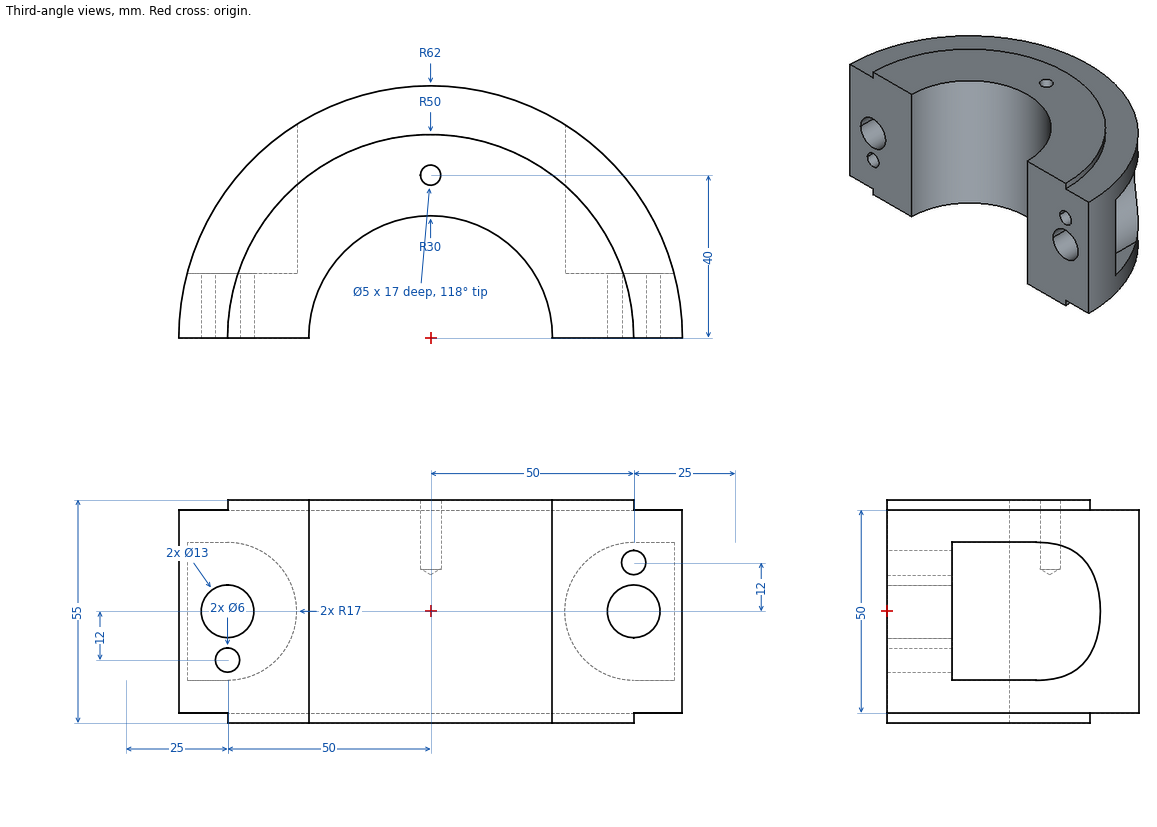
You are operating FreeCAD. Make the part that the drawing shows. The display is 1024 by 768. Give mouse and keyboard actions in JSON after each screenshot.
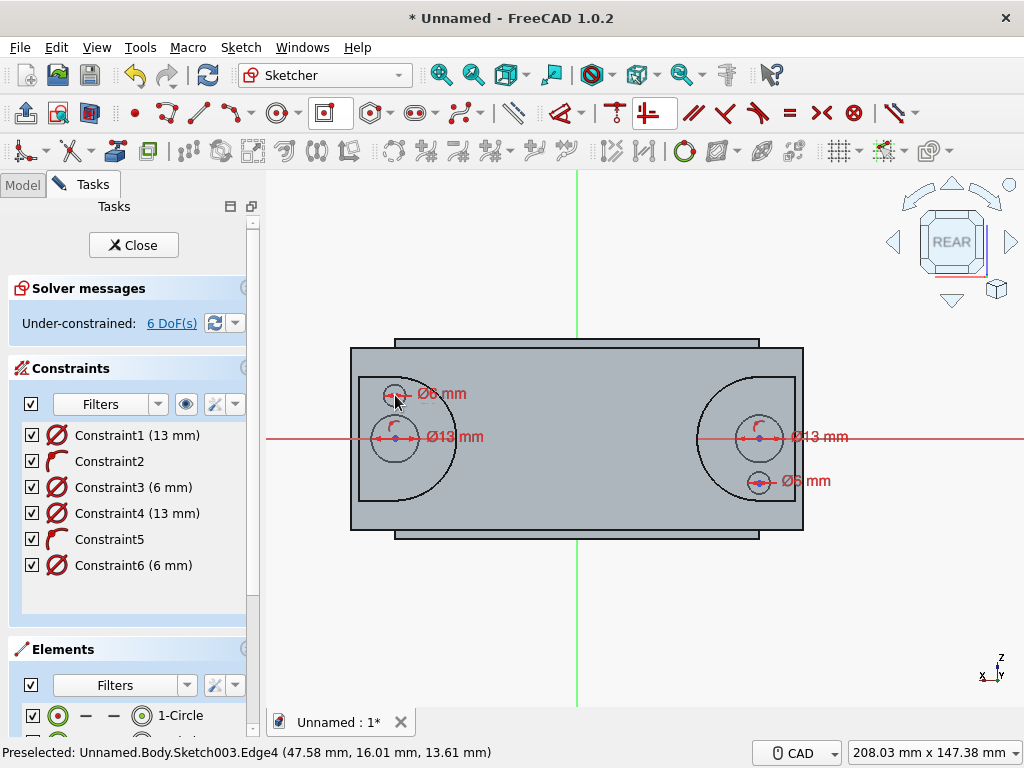
{"action": "left_click", "coordinate": [760, 439]}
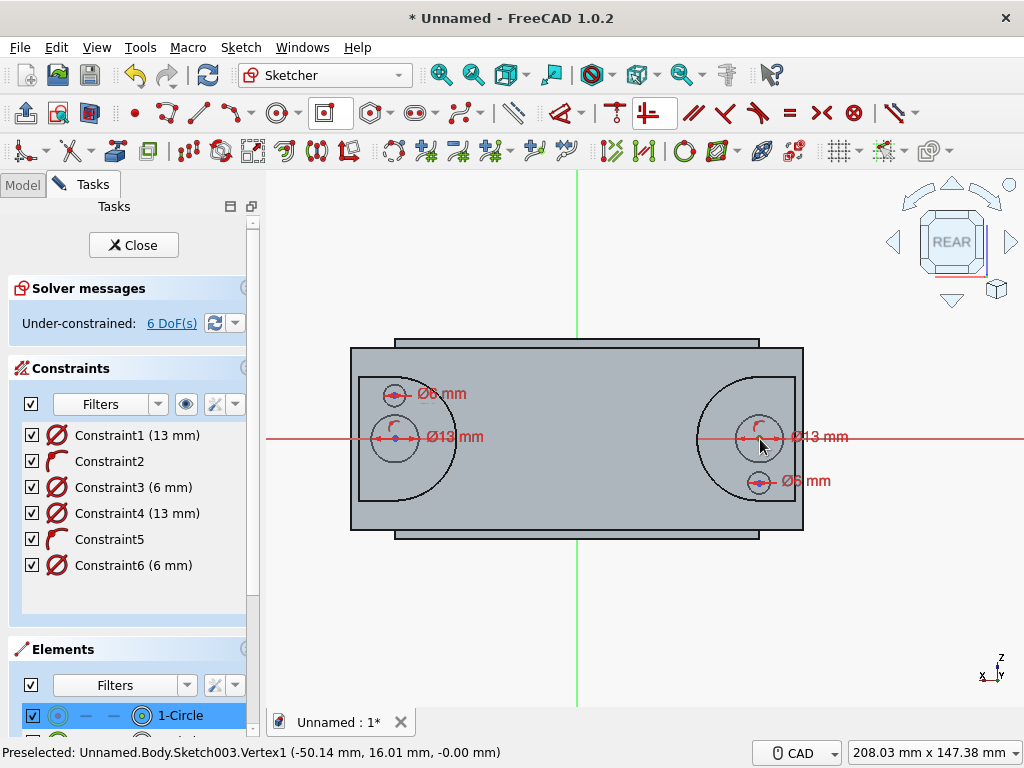
{"action": "left_click", "coordinate": [759, 483]}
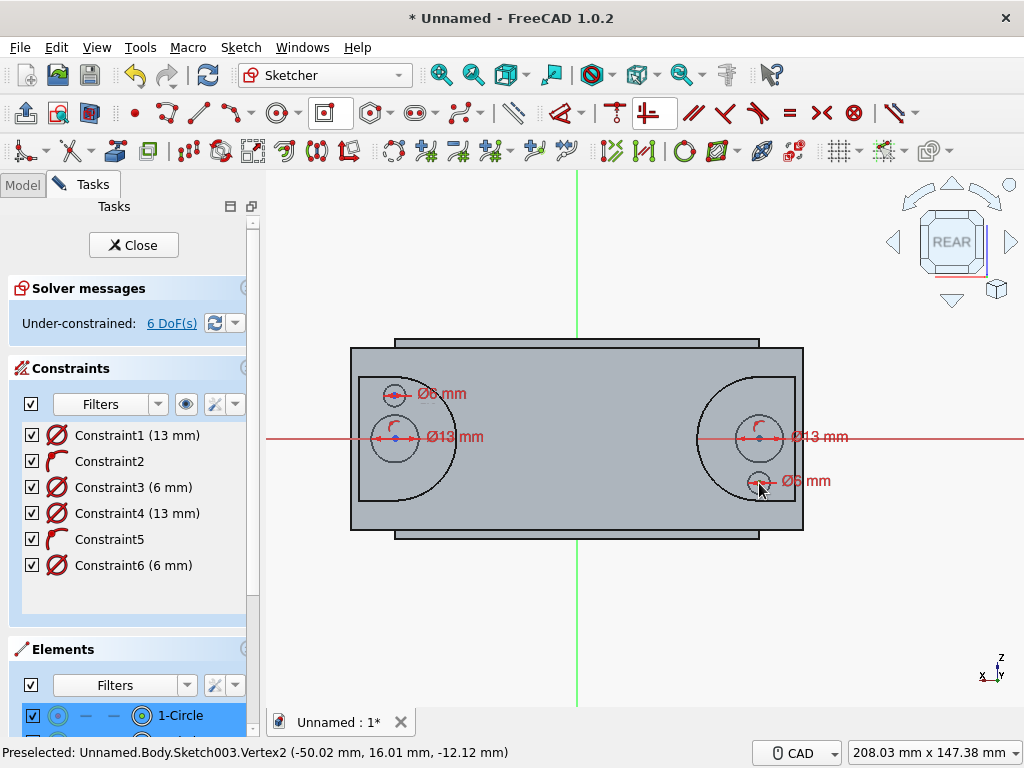
{"action": "key", "text": "v"}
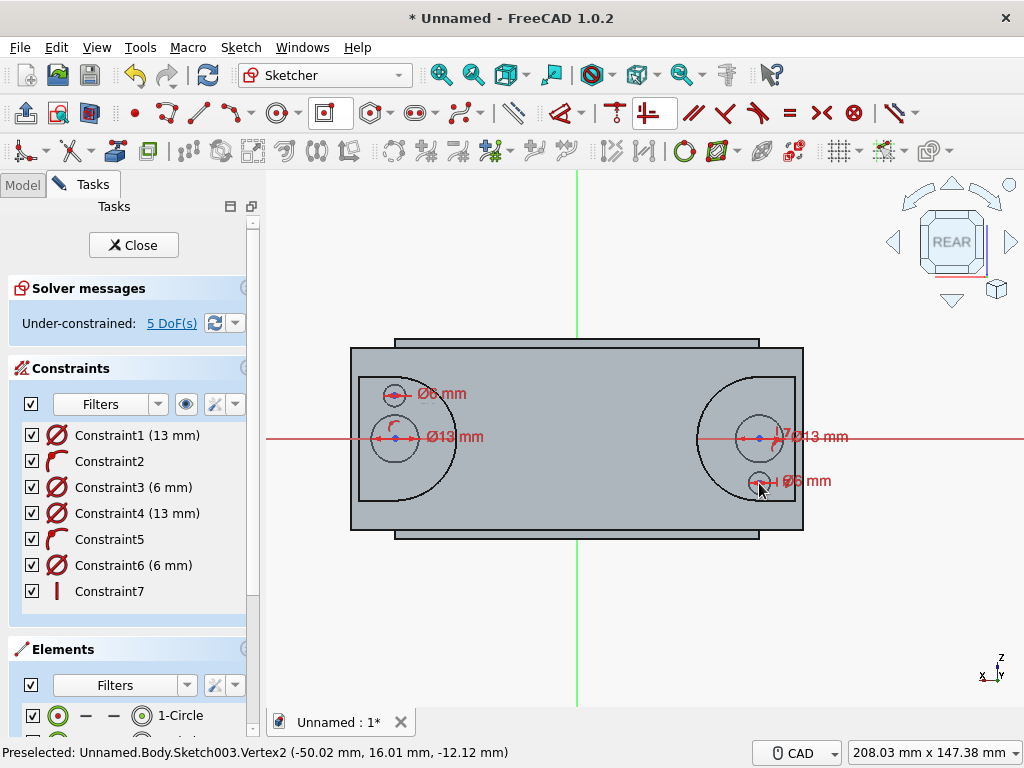
{"action": "left_click", "coordinate": [395, 439]}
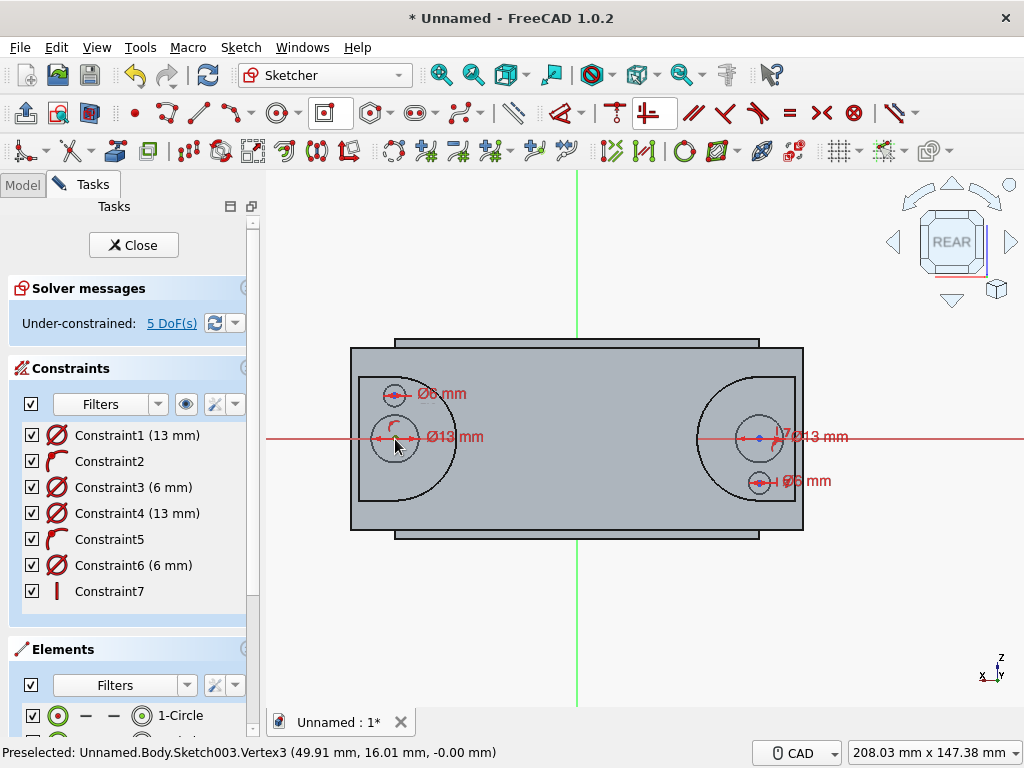
{"action": "left_click", "coordinate": [395, 396]}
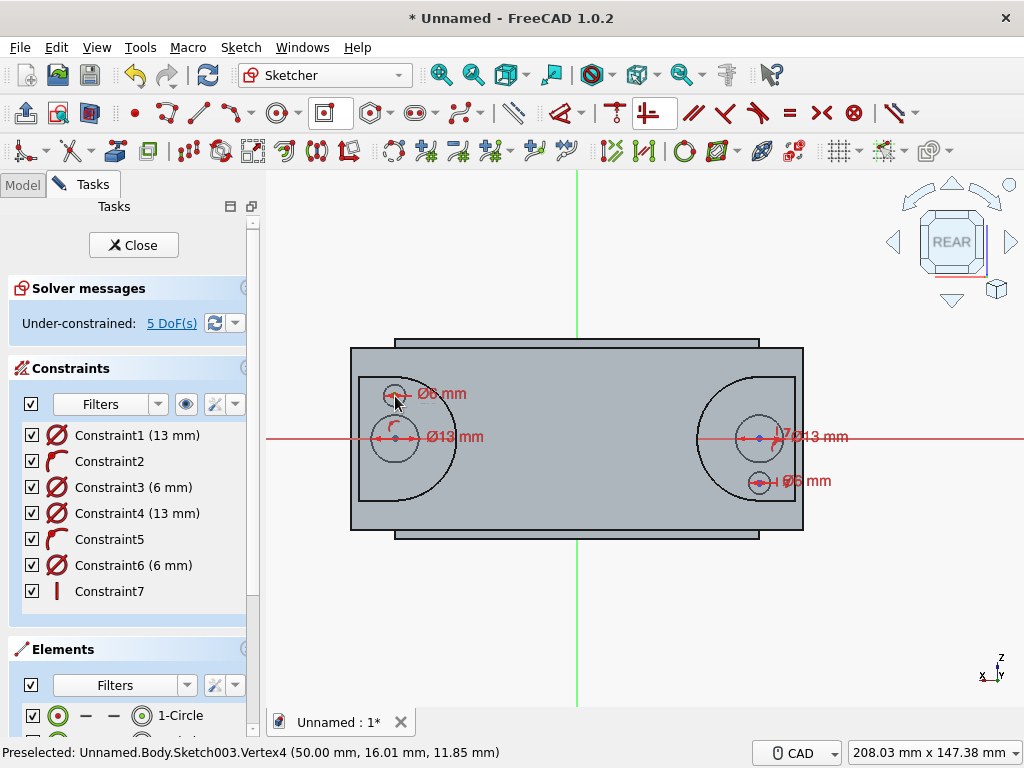
{"action": "left_click", "coordinate": [672, 114]}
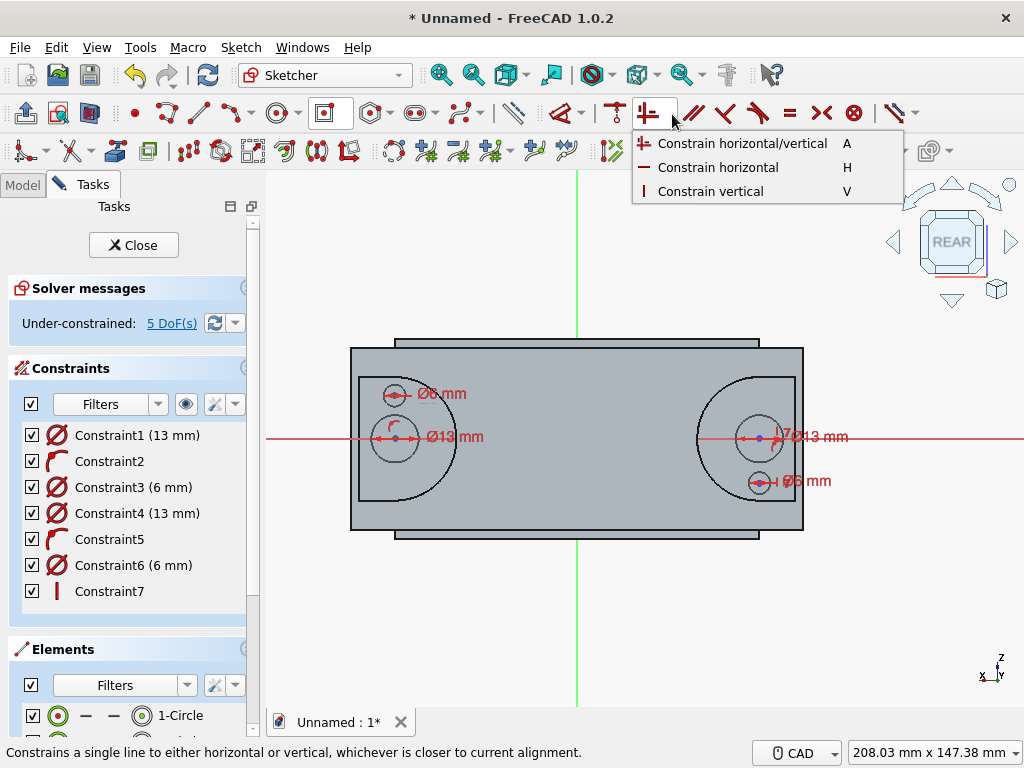
{"action": "left_click", "coordinate": [768, 191]}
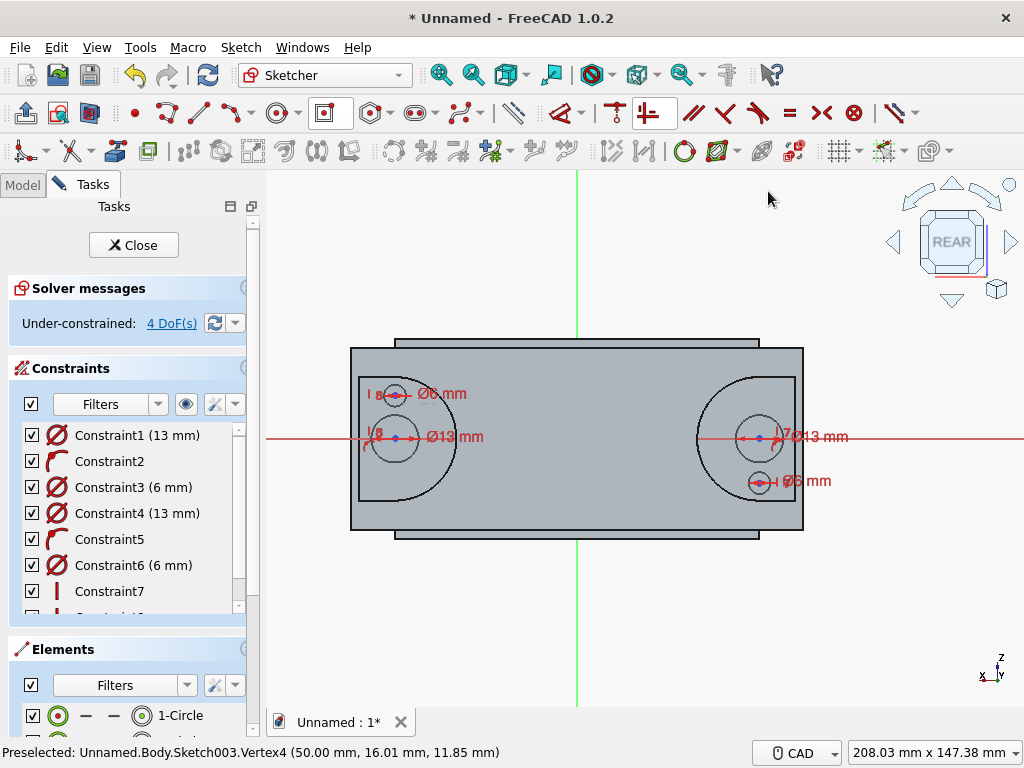
{"action": "left_click", "coordinate": [560, 114]}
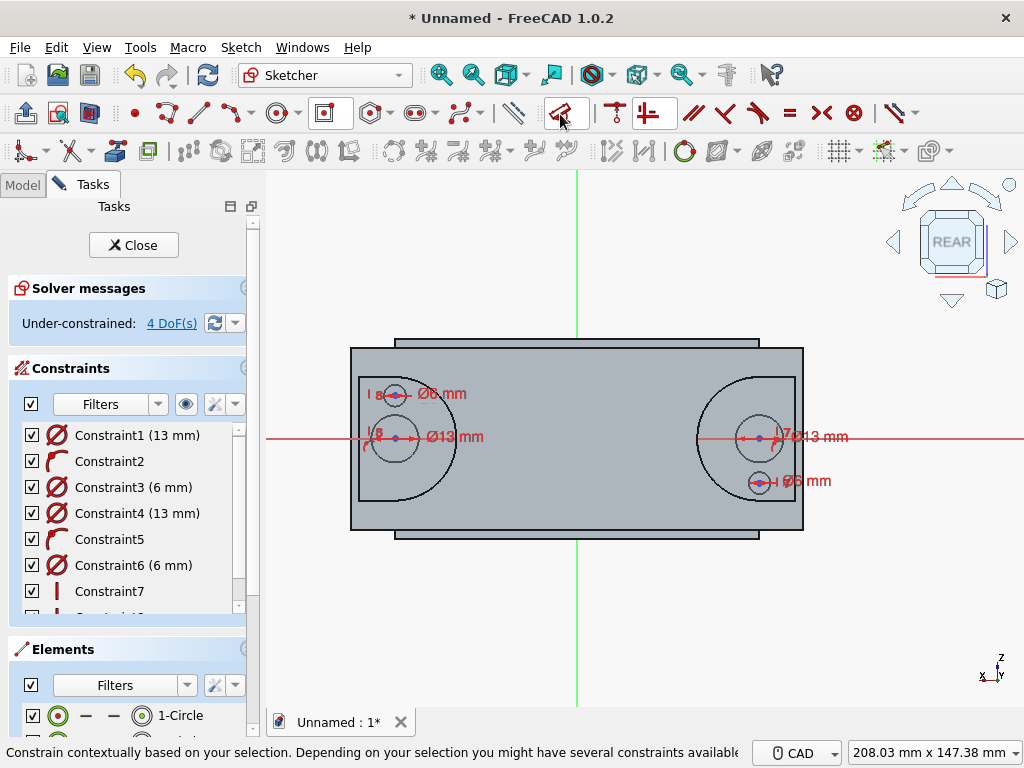
{"action": "left_click", "coordinate": [760, 439]}
{"action": "left_click", "coordinate": [668, 473]}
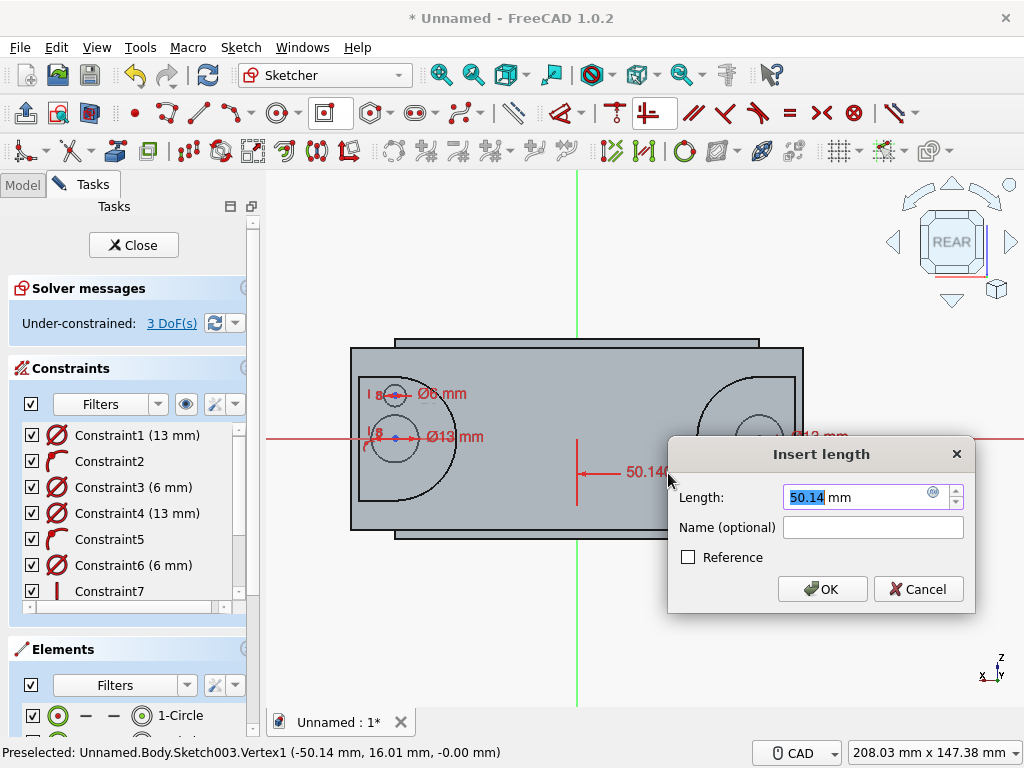
{"action": "type", "text": "50"}
{"action": "key", "text": "Return"}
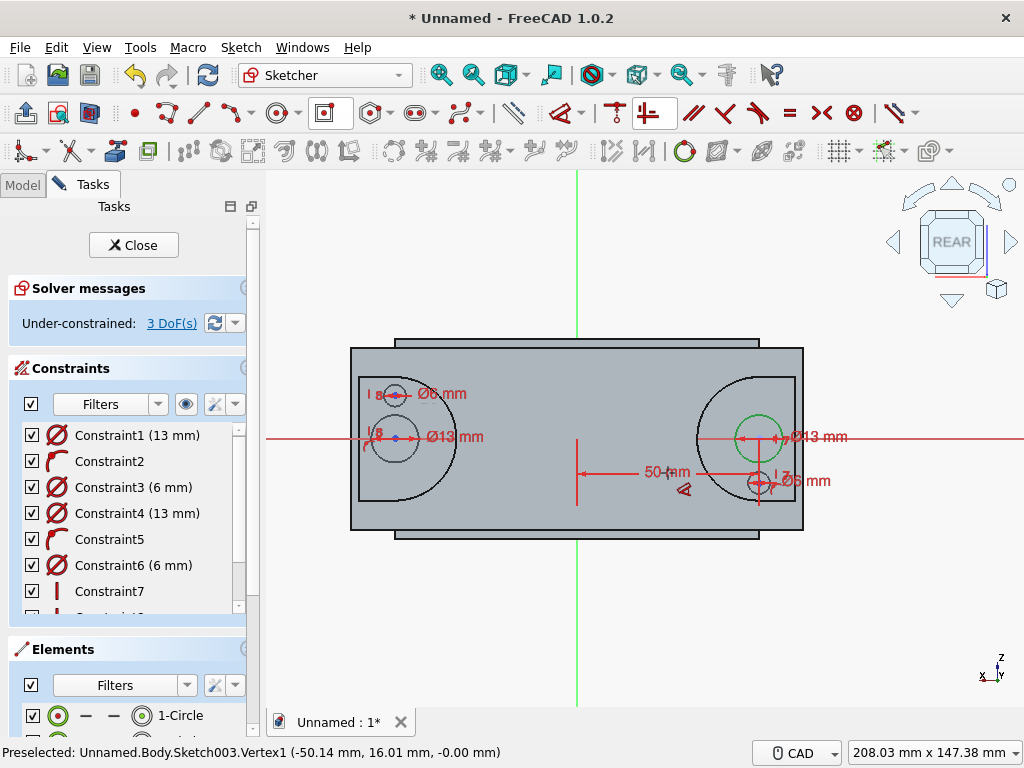
{"action": "left_click", "coordinate": [759, 483]}
{"action": "left_click", "coordinate": [793, 461]}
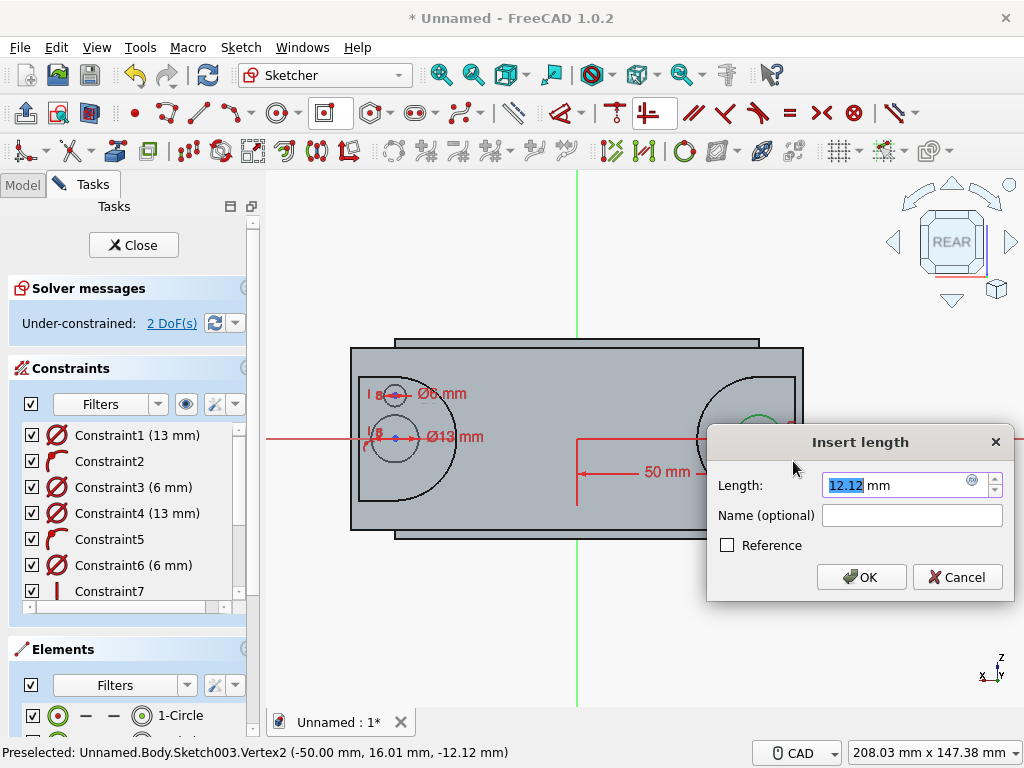
{"action": "type", "text": "12"}
{"action": "key", "text": "Return"}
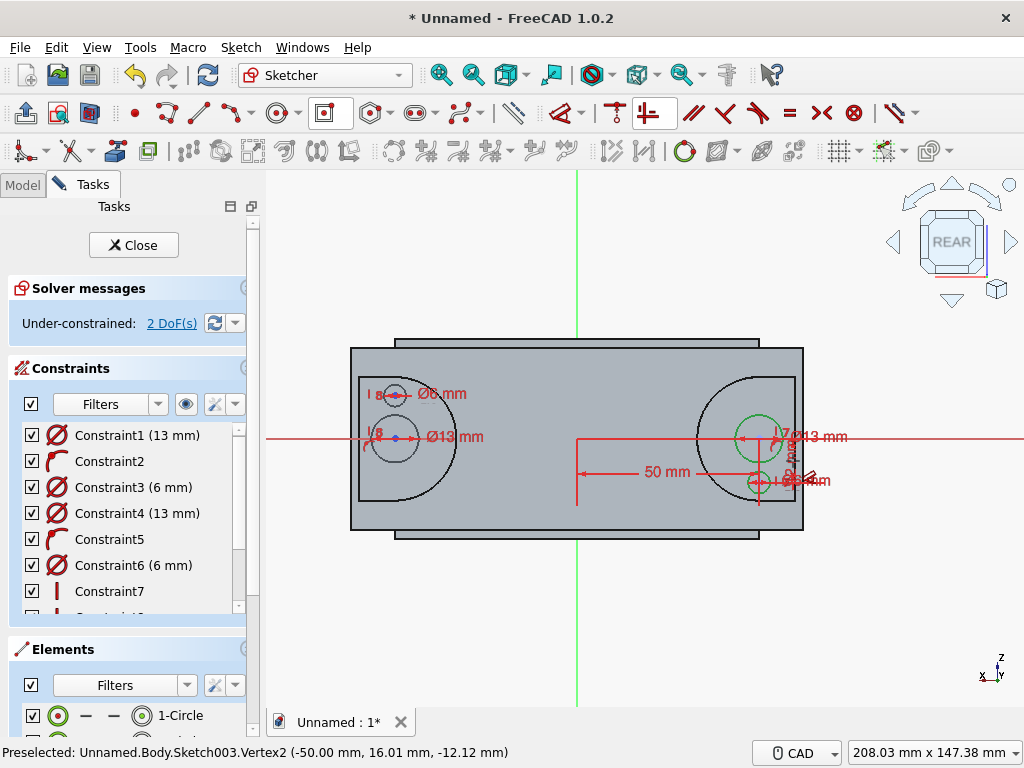
{"action": "left_click", "coordinate": [395, 439]}
{"action": "left_click", "coordinate": [486, 473]}